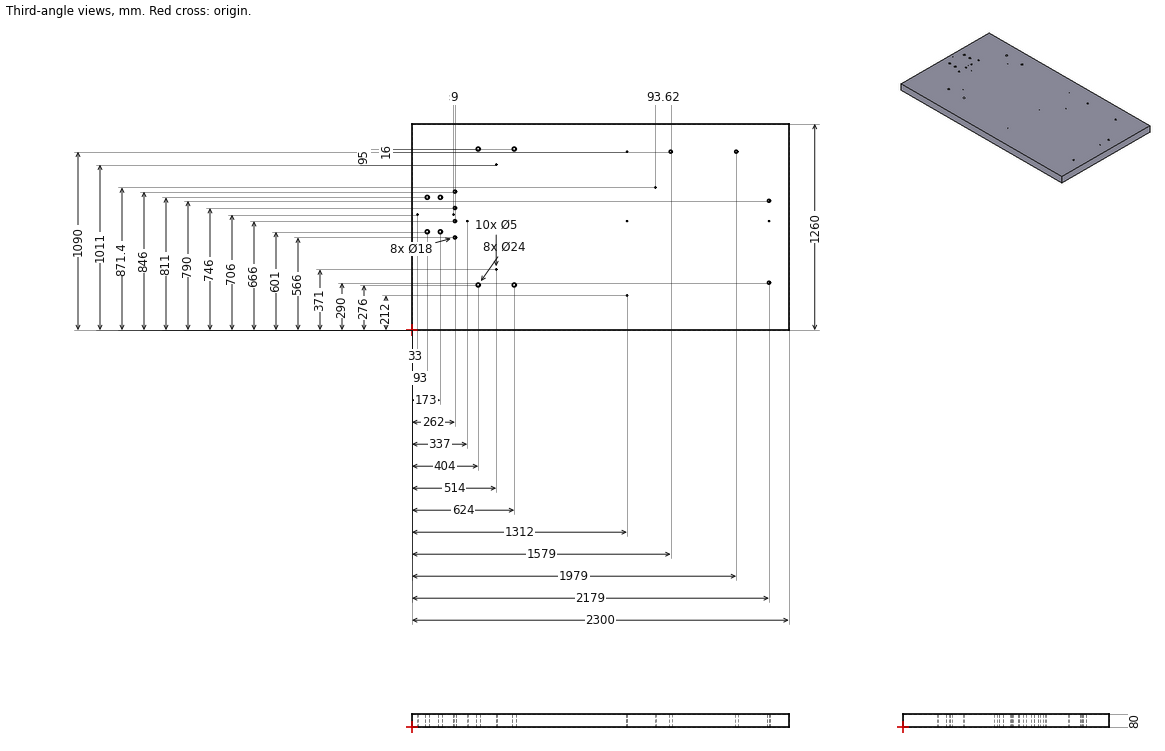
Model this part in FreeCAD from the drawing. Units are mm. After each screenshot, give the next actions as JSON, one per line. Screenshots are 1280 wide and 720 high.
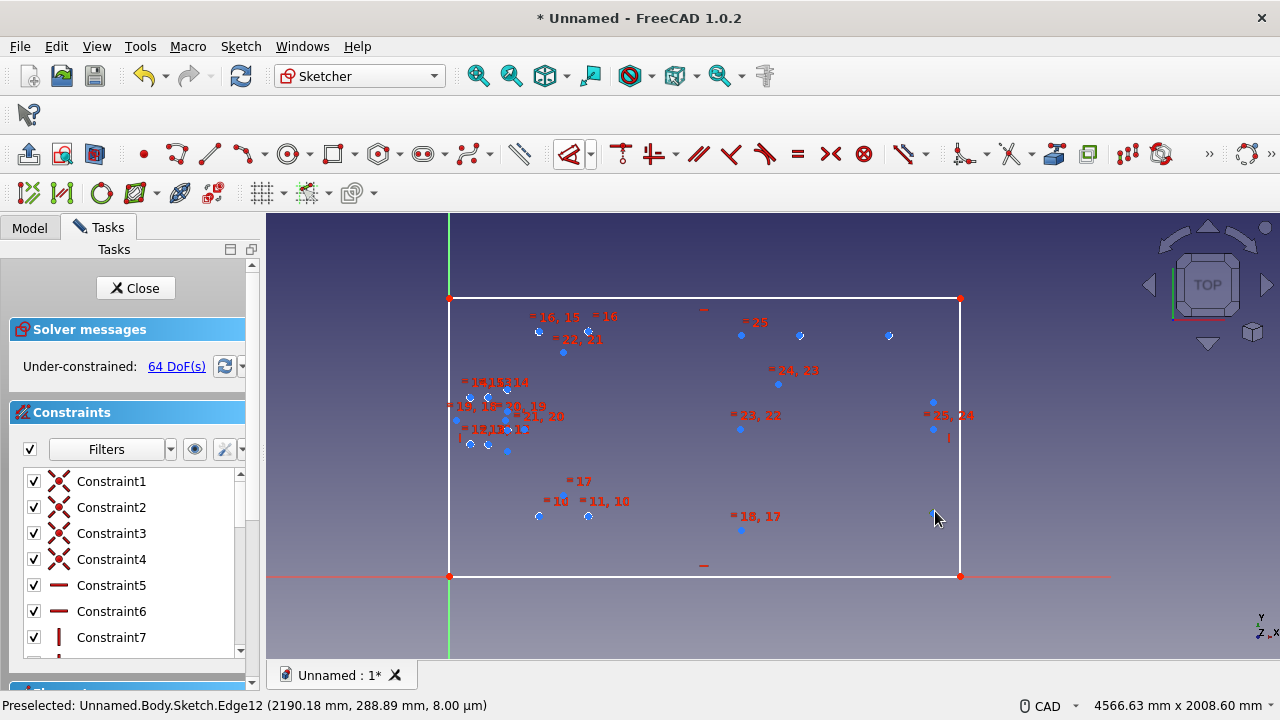
{"action": "scroll", "coordinate": [510, 428], "scroll_direction": "up", "scroll_amount": 8}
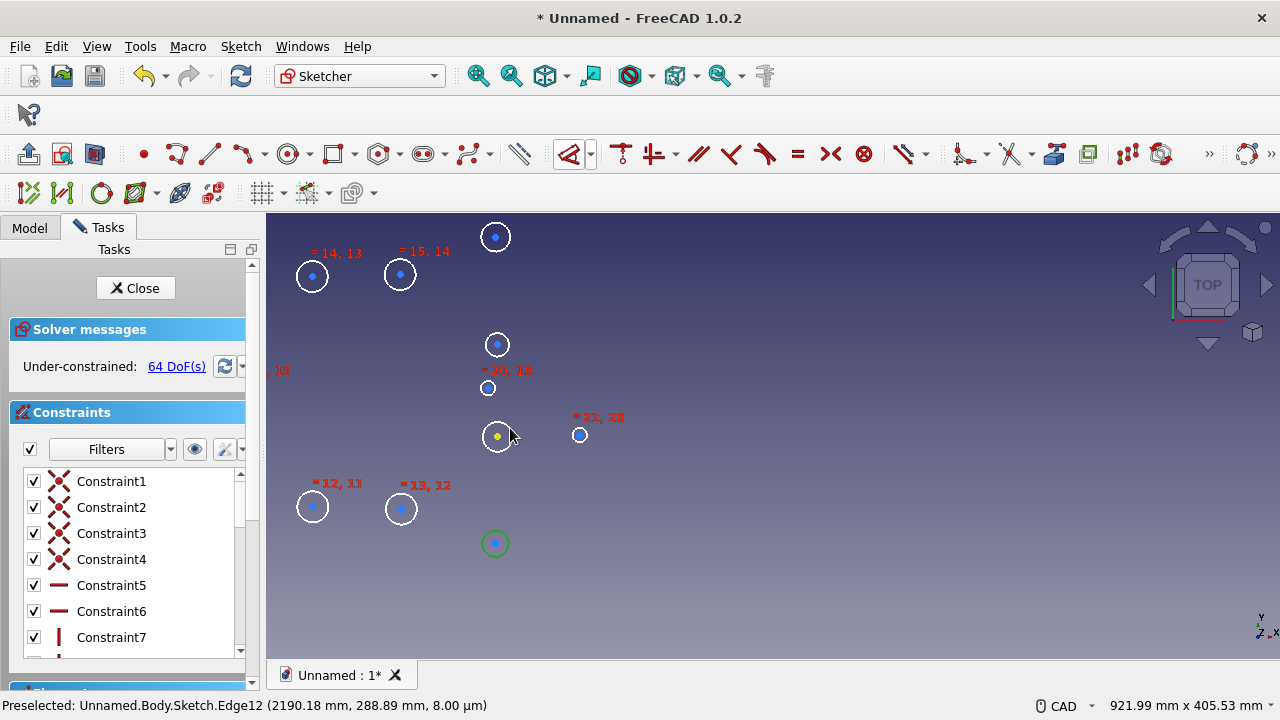
{"action": "left_click", "coordinate": [508, 426]}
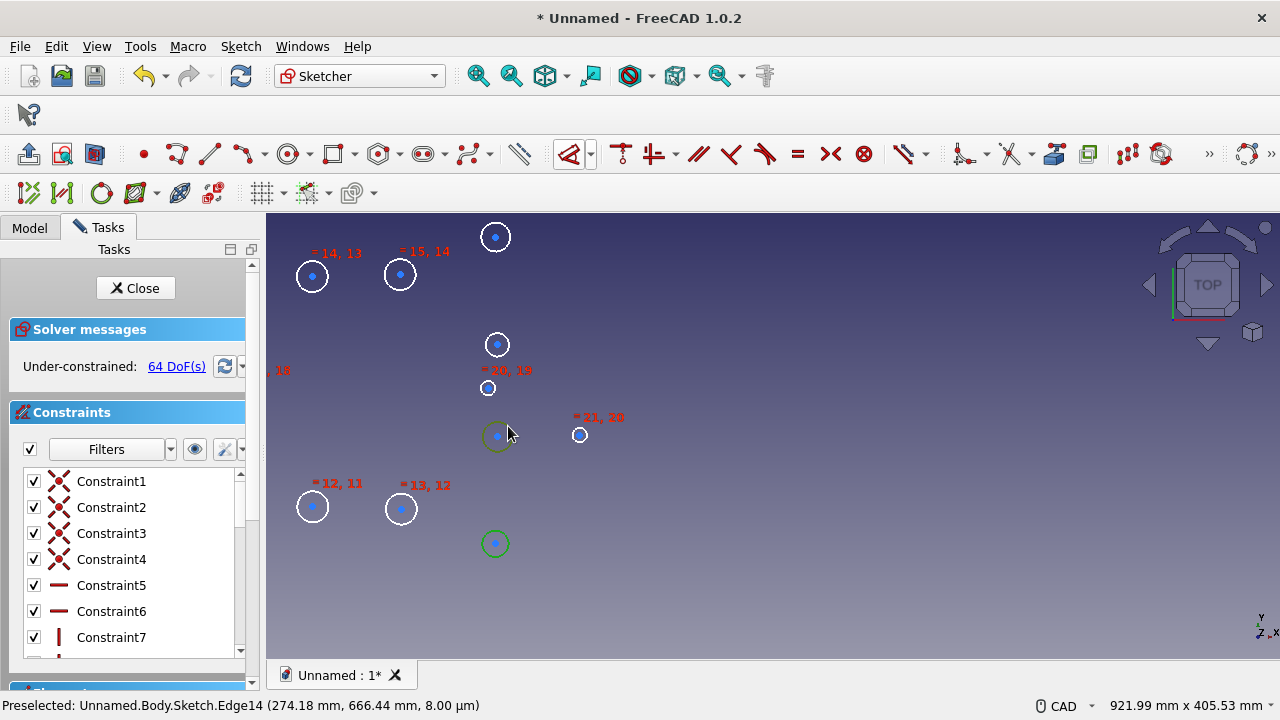
{"action": "left_click", "coordinate": [506, 337]}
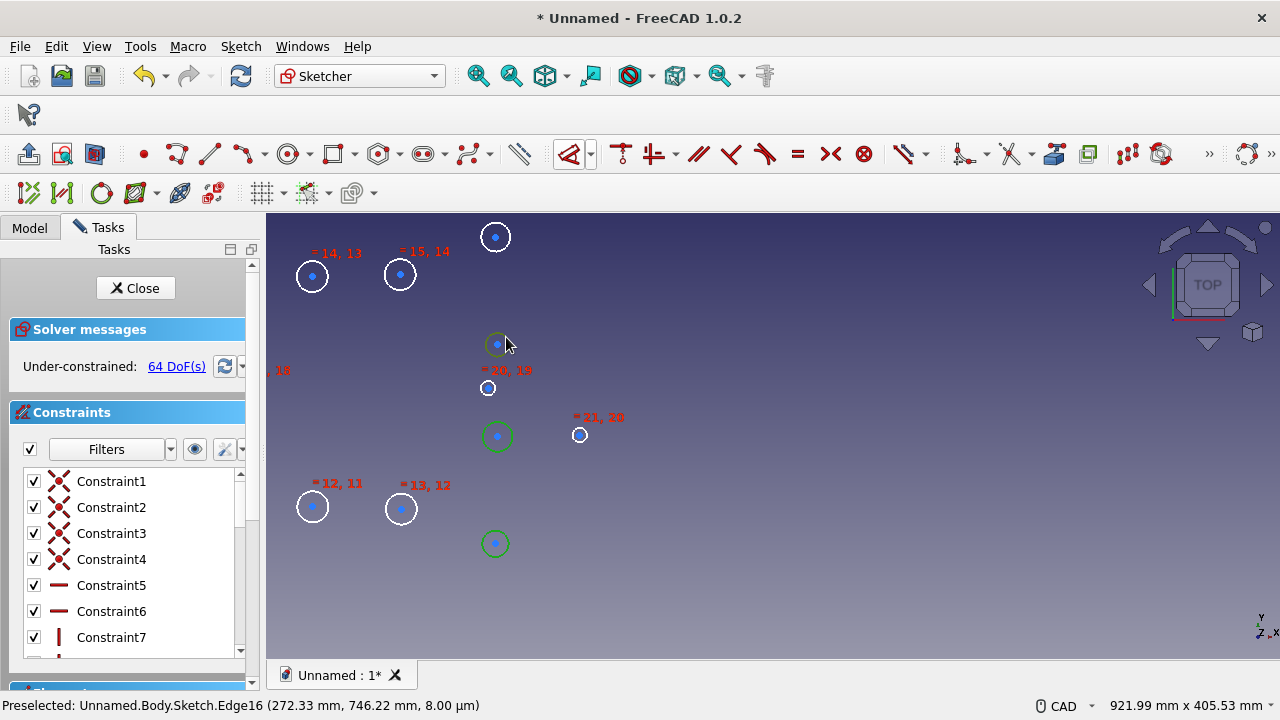
{"action": "left_click", "coordinate": [486, 247]}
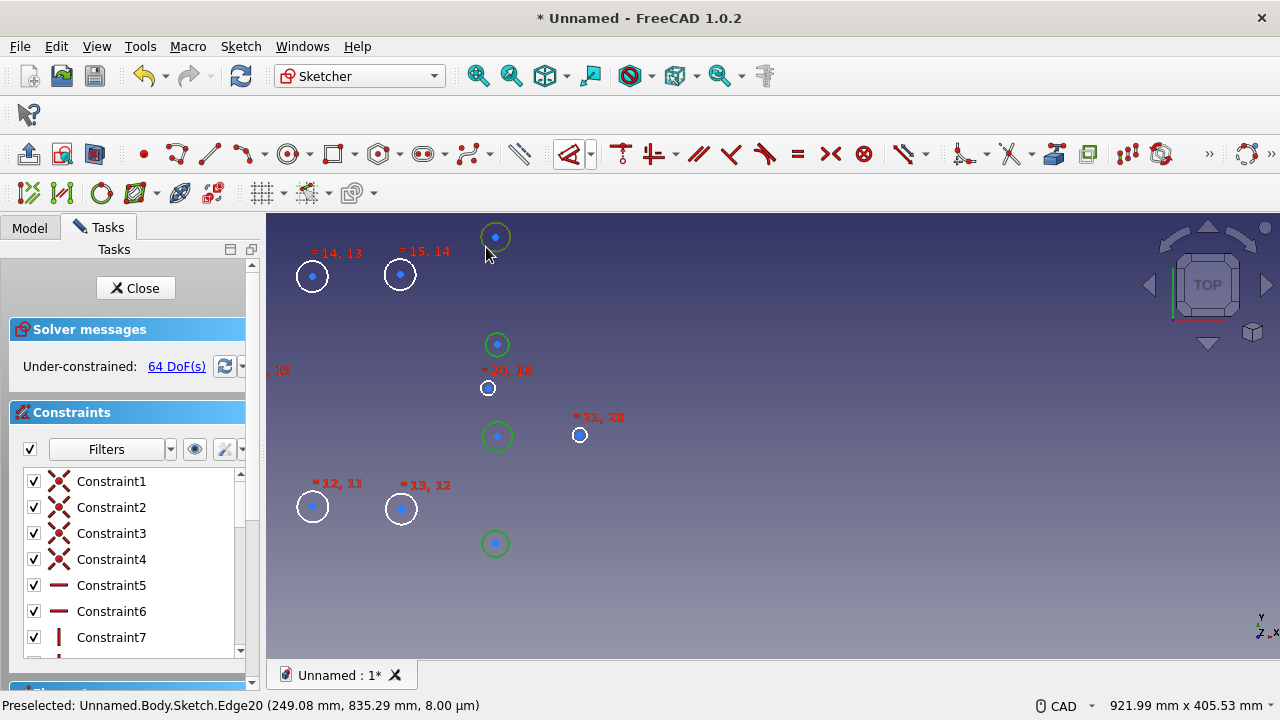
{"action": "scroll", "coordinate": [510, 427], "scroll_direction": "down", "scroll_amount": 8}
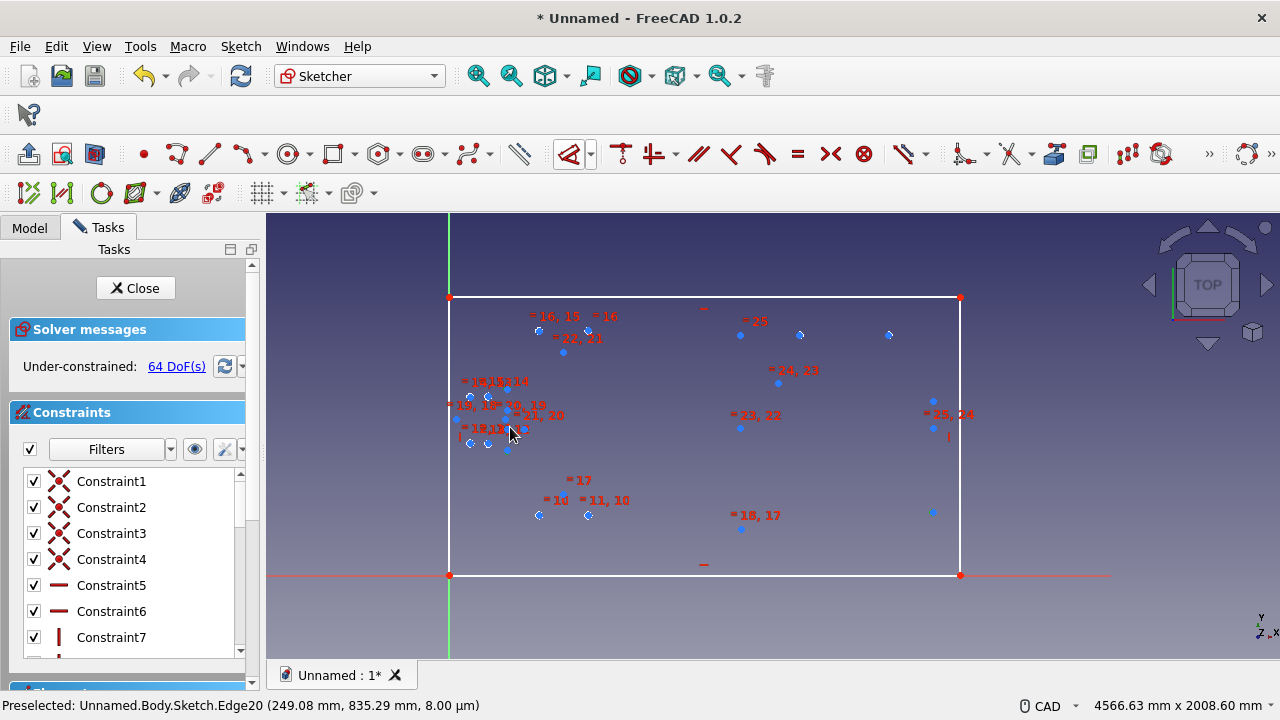
{"action": "scroll", "coordinate": [935, 400], "scroll_direction": "up", "scroll_amount": 9}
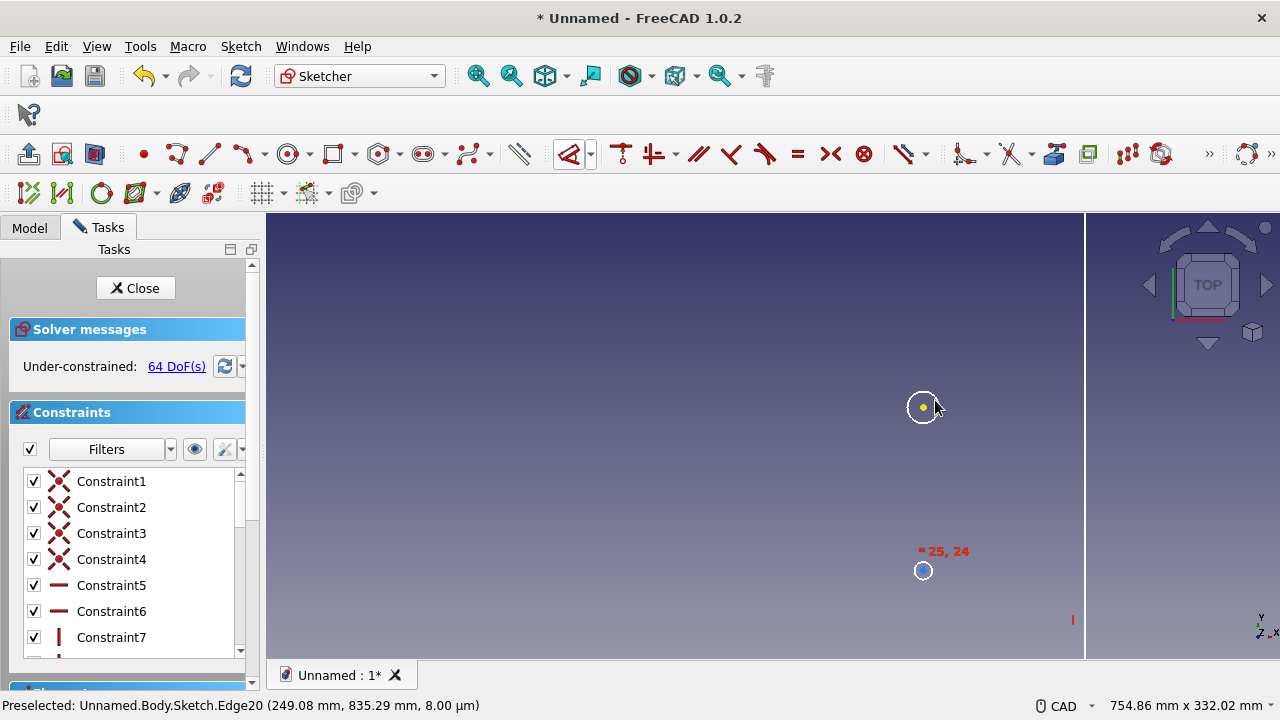
{"action": "left_click", "coordinate": [934, 396]}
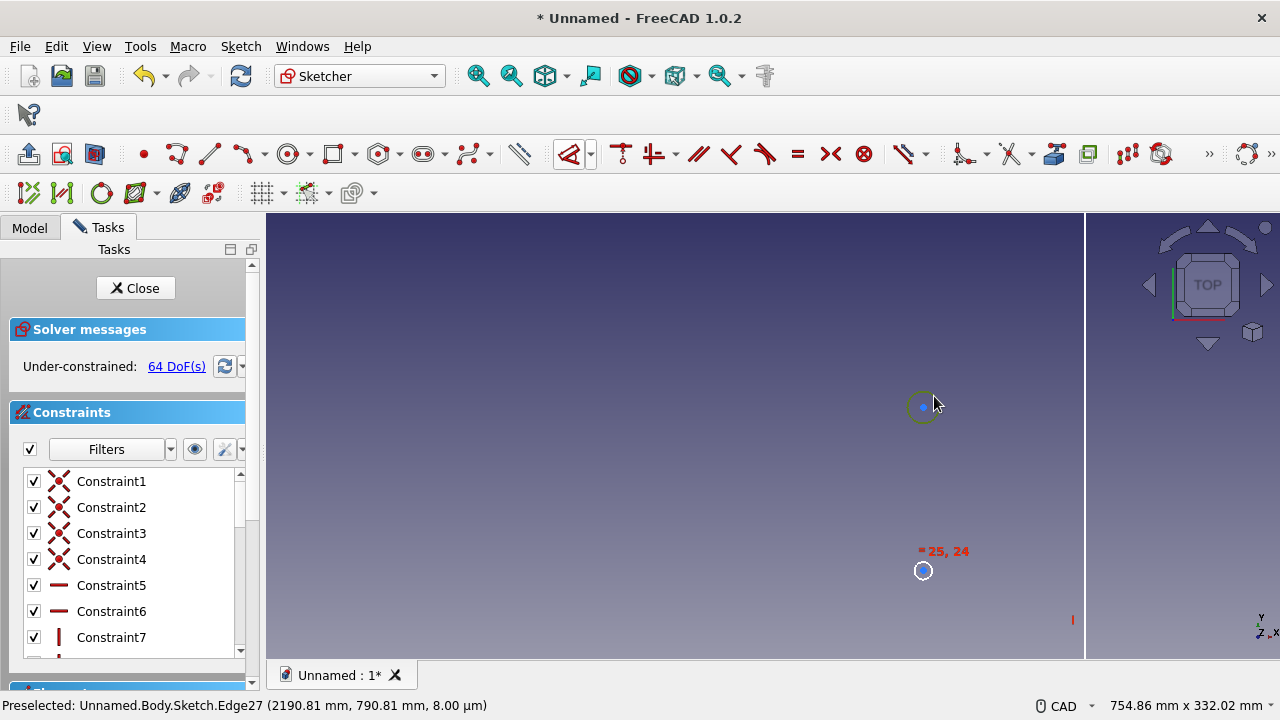
{"action": "scroll", "coordinate": [935, 400], "scroll_direction": "down", "scroll_amount": 9}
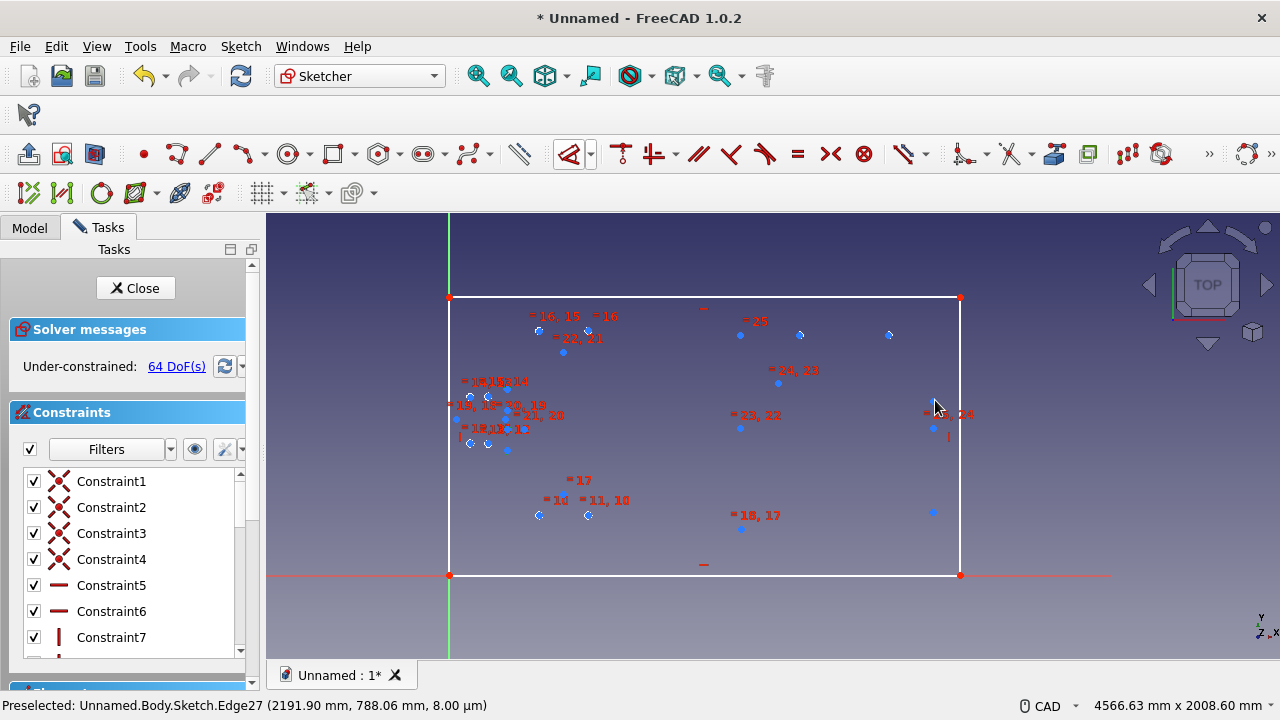
{"action": "scroll", "coordinate": [802, 333], "scroll_direction": "up", "scroll_amount": 8}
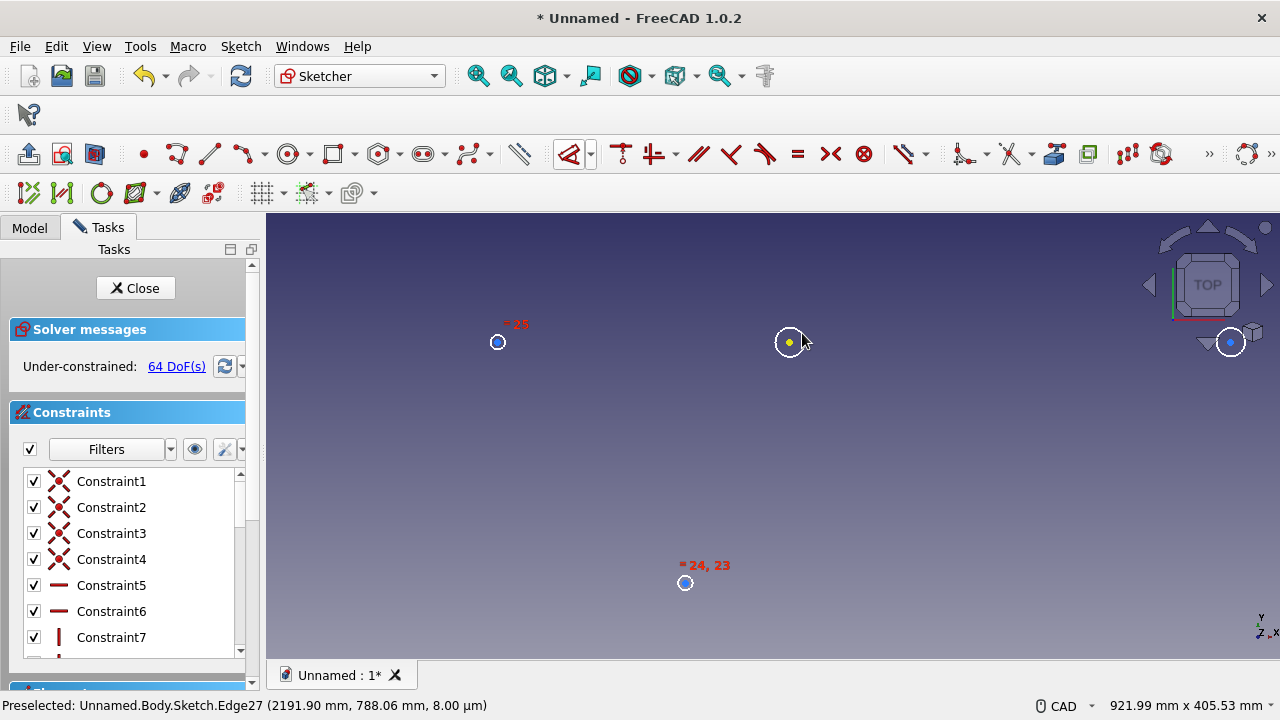
{"action": "left_click", "coordinate": [800, 332]}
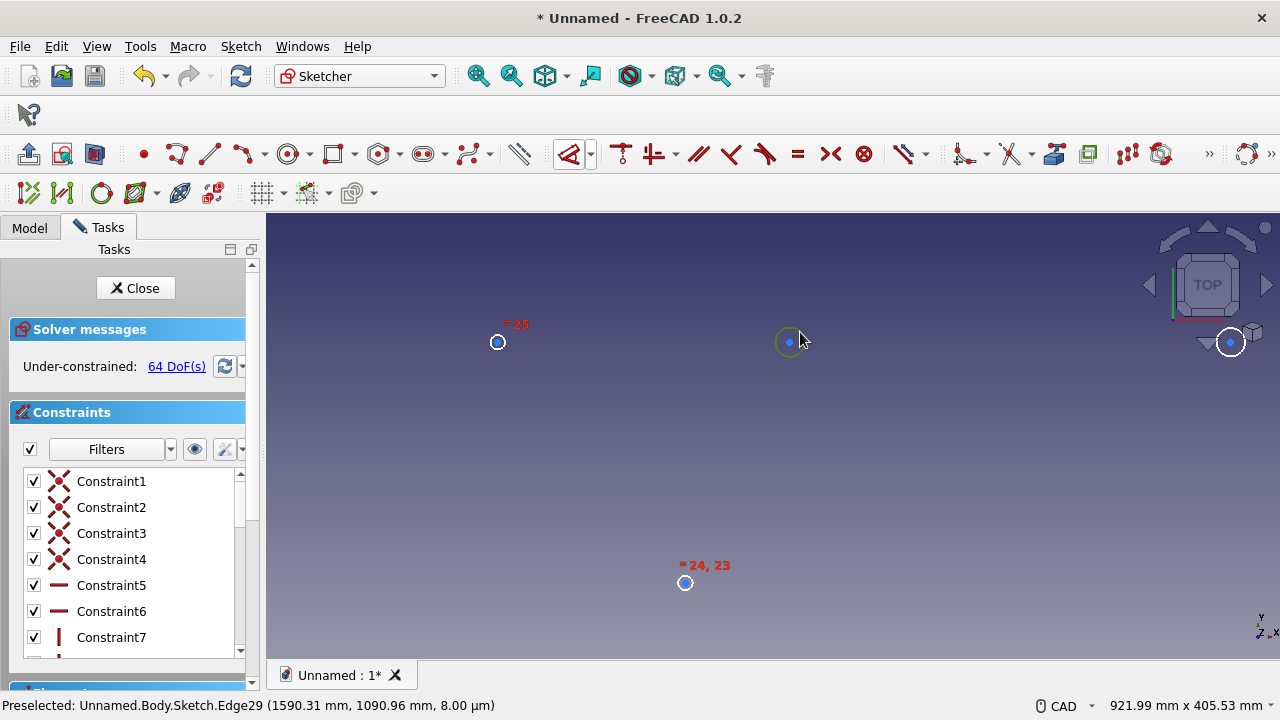
{"action": "scroll", "coordinate": [802, 333], "scroll_direction": "down", "scroll_amount": 8}